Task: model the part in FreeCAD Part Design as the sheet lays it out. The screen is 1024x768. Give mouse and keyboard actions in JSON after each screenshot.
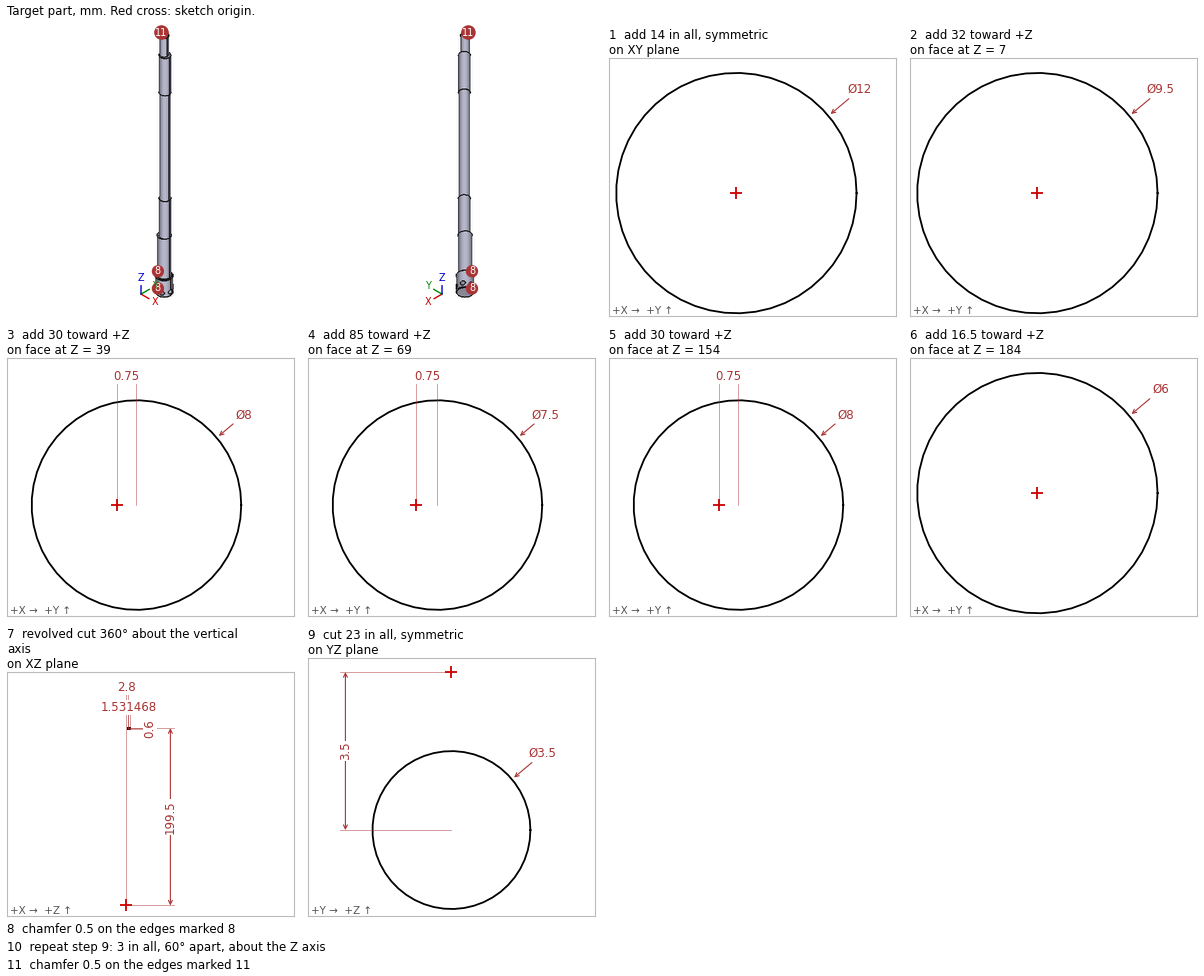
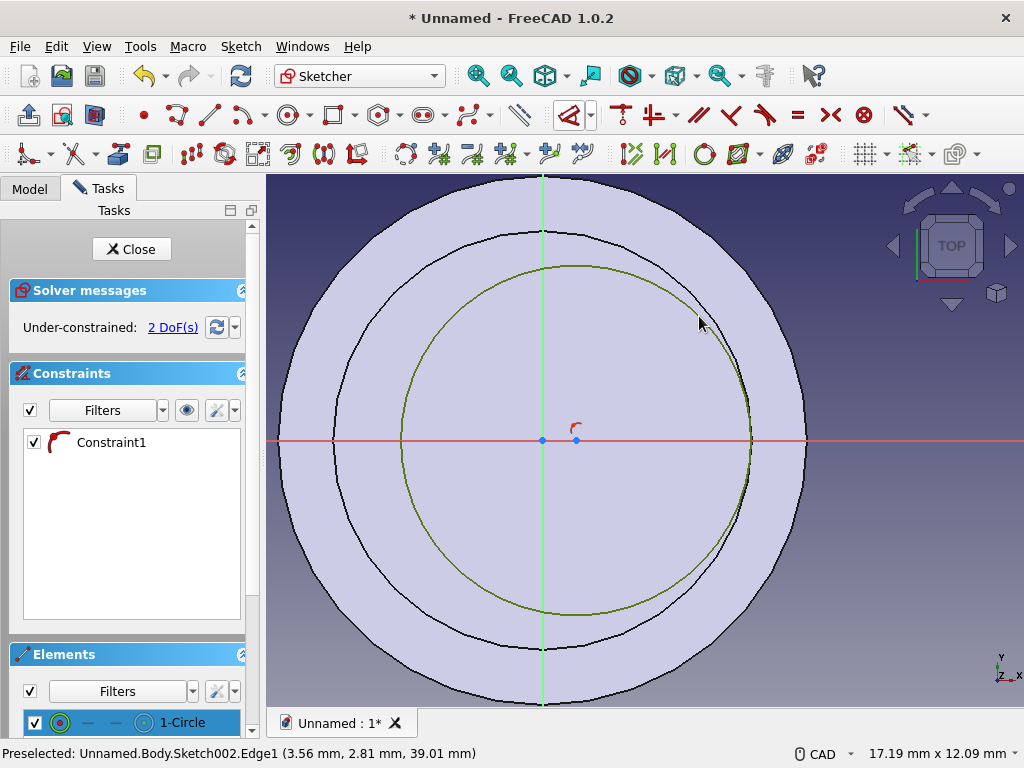
{"action": "key", "text": "k o"}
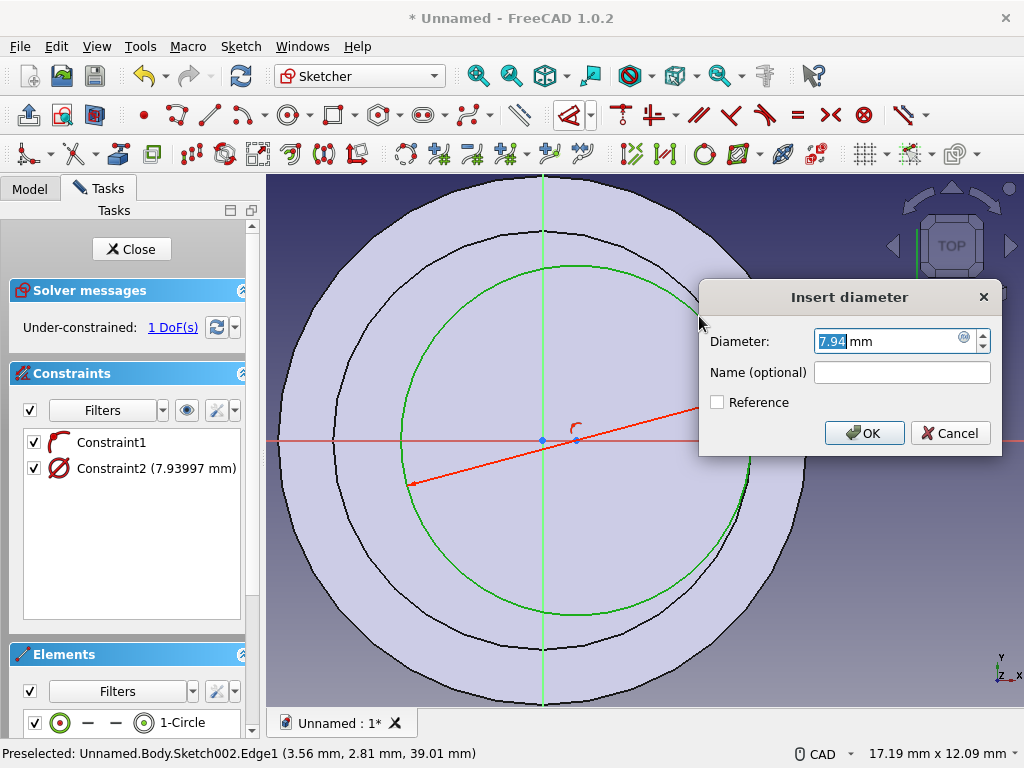
{"action": "type", "text": "8"}
{"action": "key", "text": "Return"}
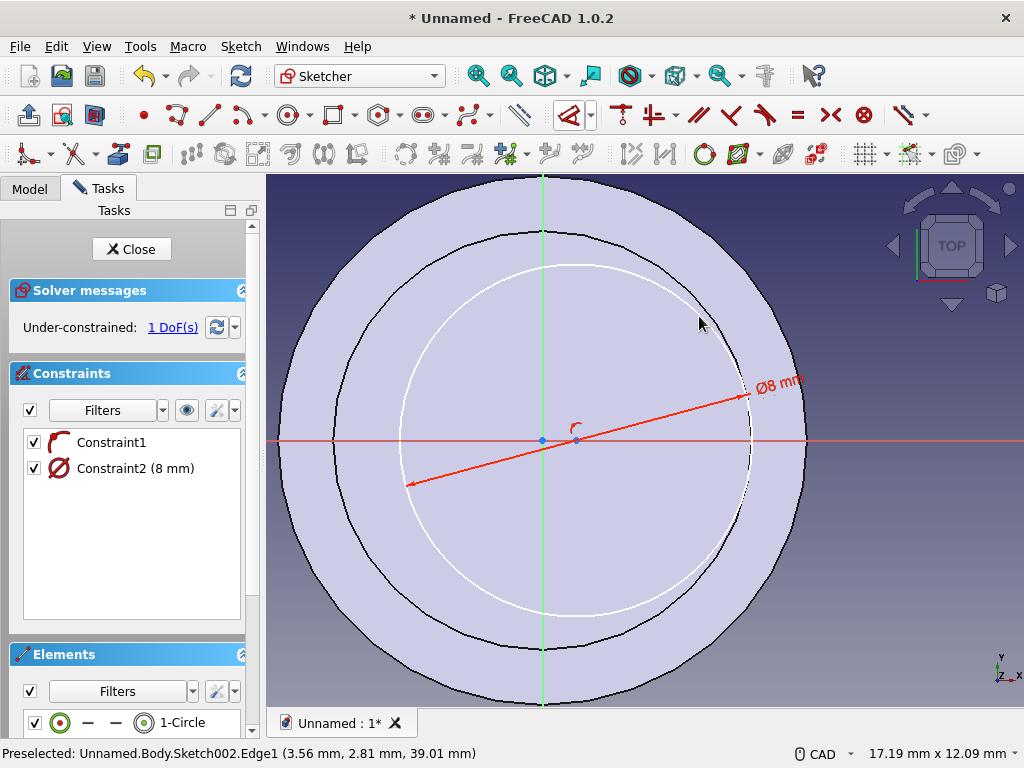
{"action": "left_click", "coordinate": [576, 440]}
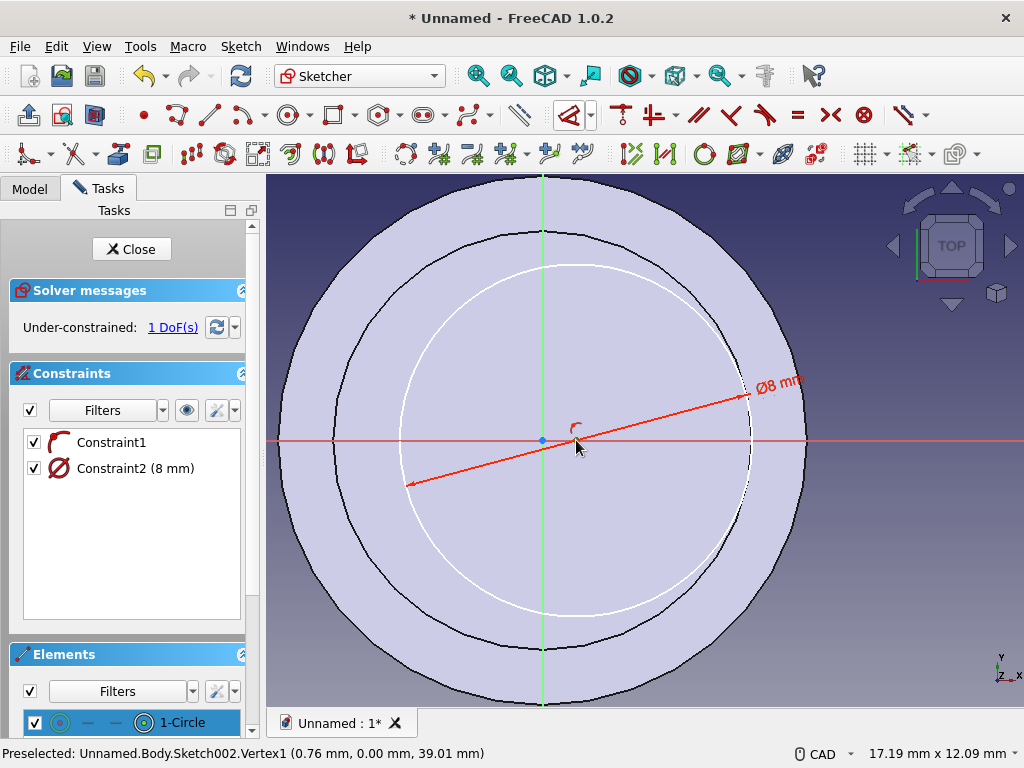
{"action": "key", "text": "l"}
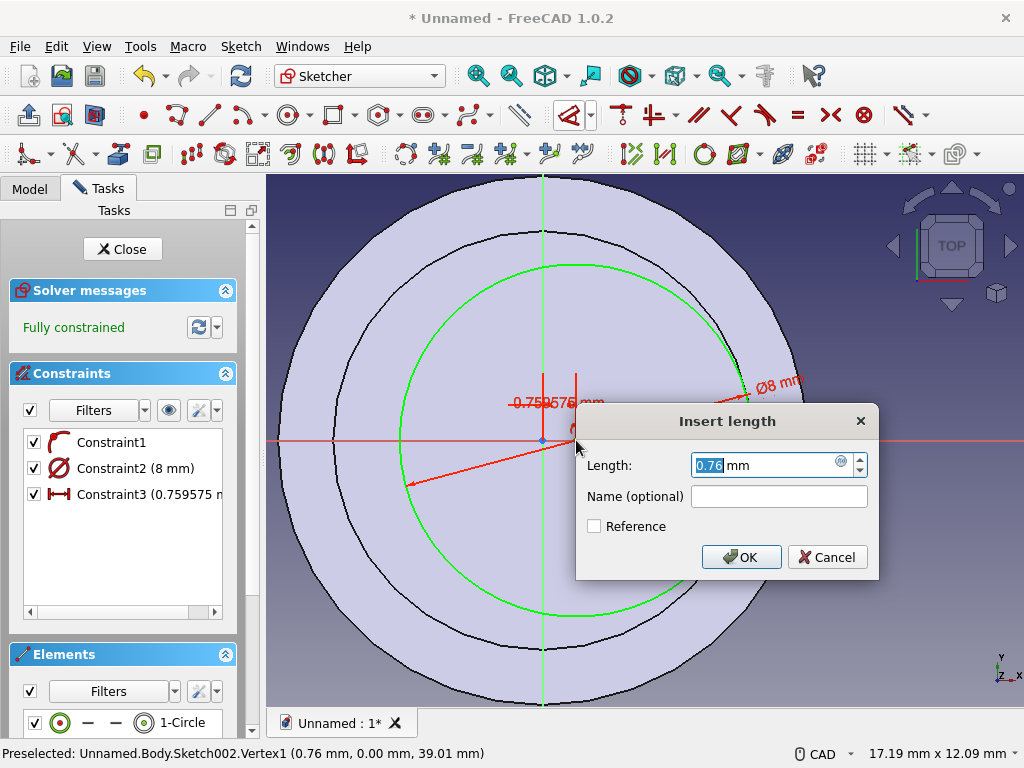
{"action": "type", "text": "0.75"}
{"action": "key", "text": "Return"}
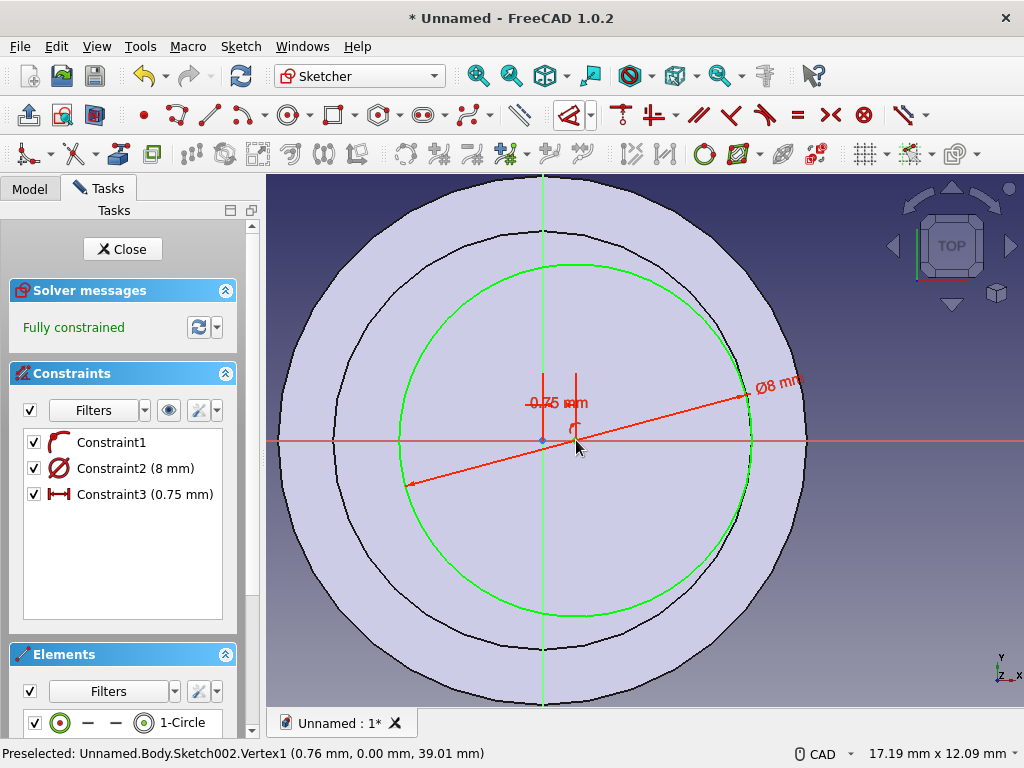
{"action": "left_click", "coordinate": [123, 249]}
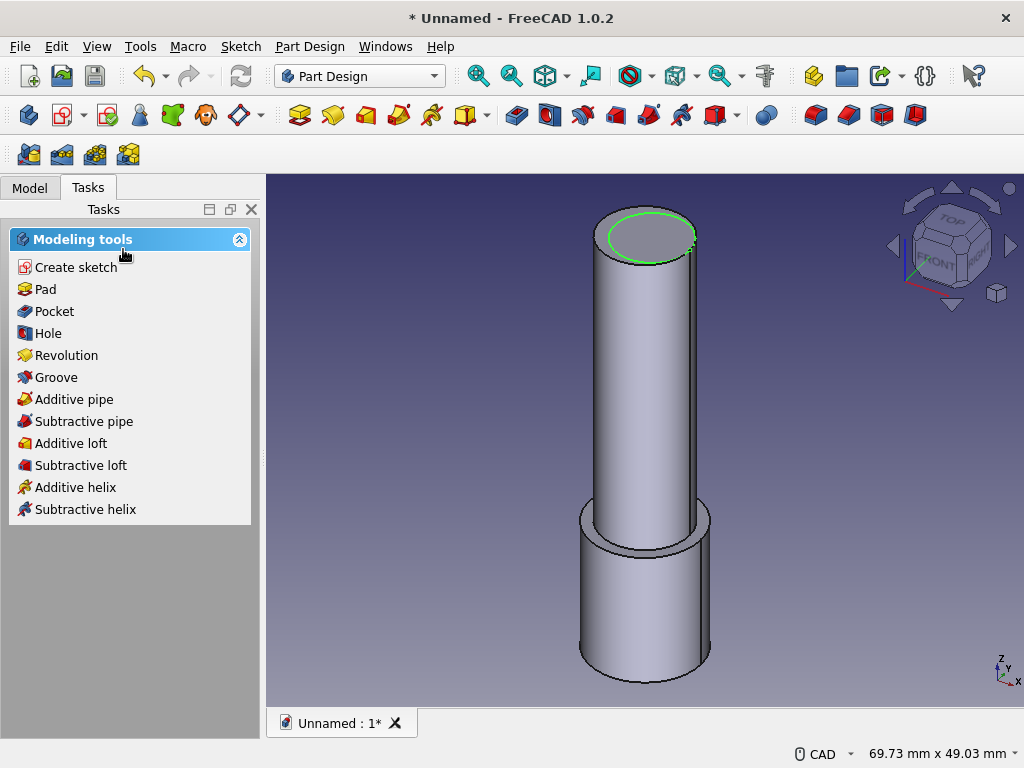
{"action": "left_click", "coordinate": [300, 116]}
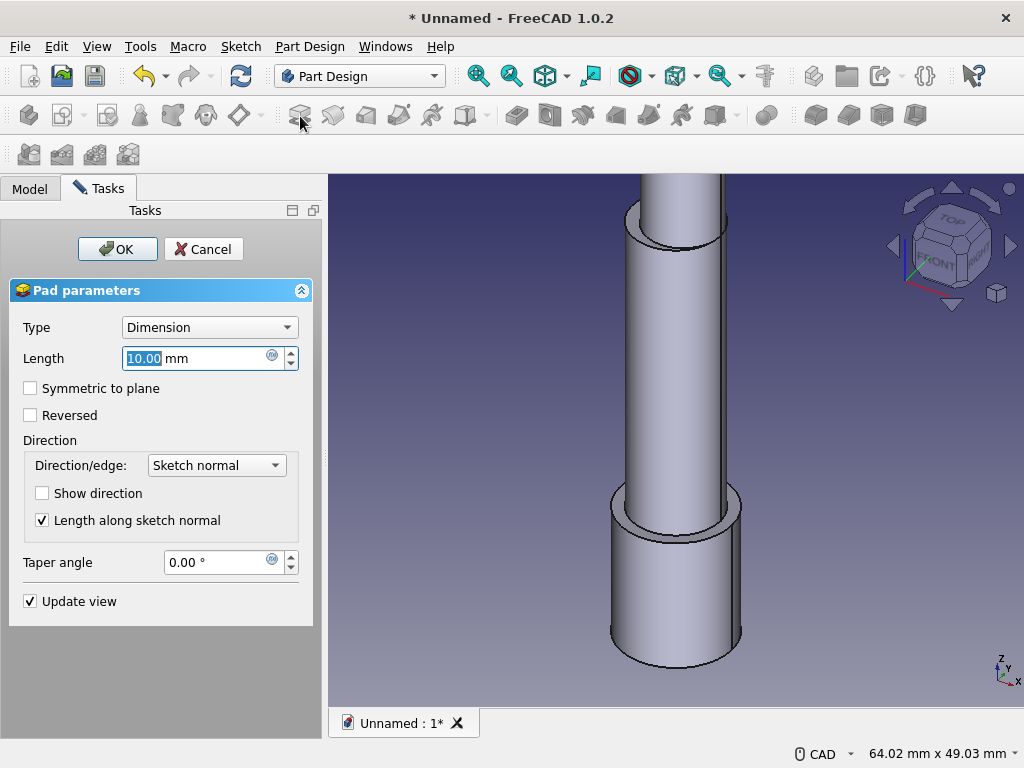
{"action": "type", "text": "30"}
{"action": "key", "text": "Tab"}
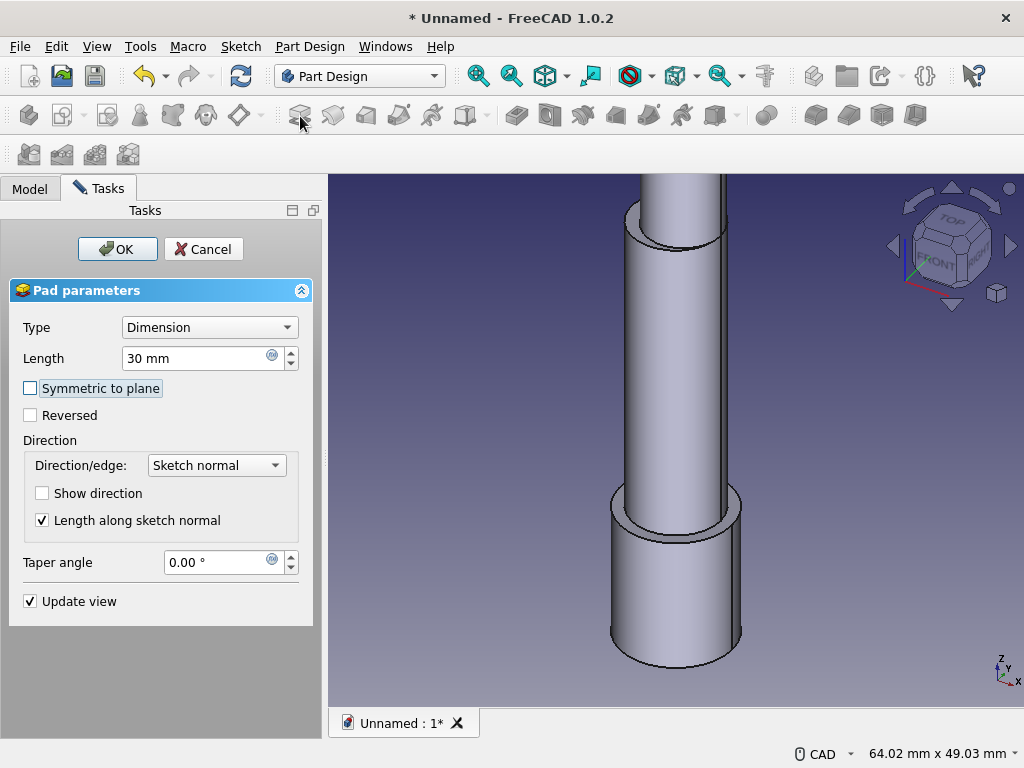
{"action": "left_click", "coordinate": [118, 249]}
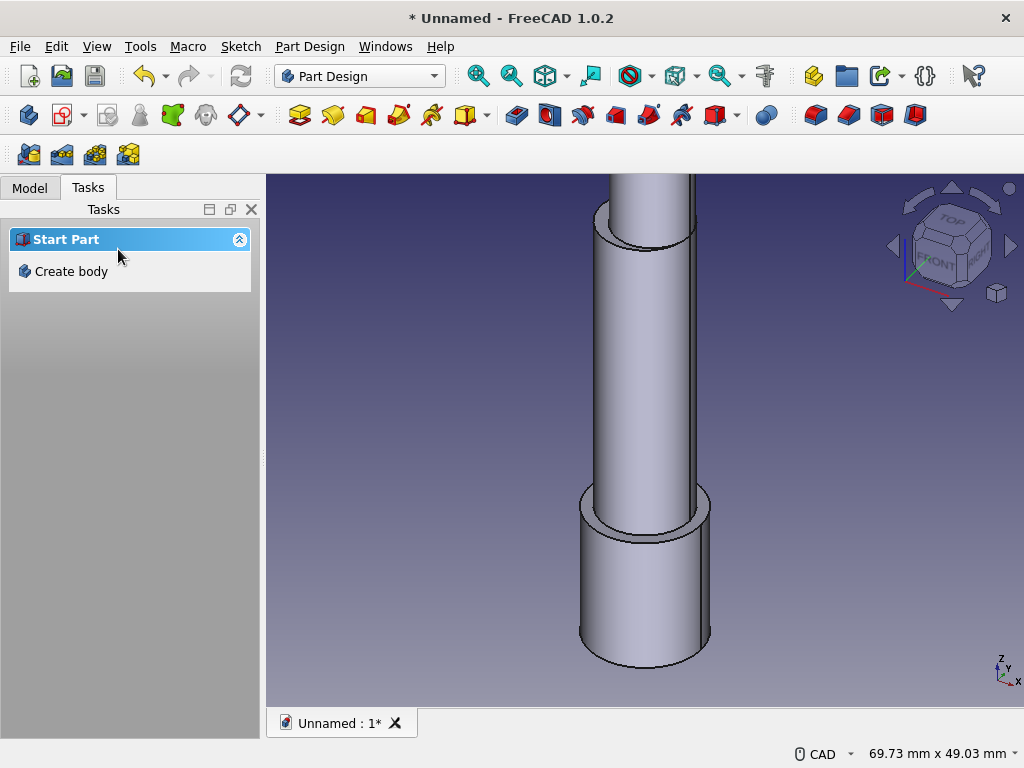
{"action": "key", "text": "v f"}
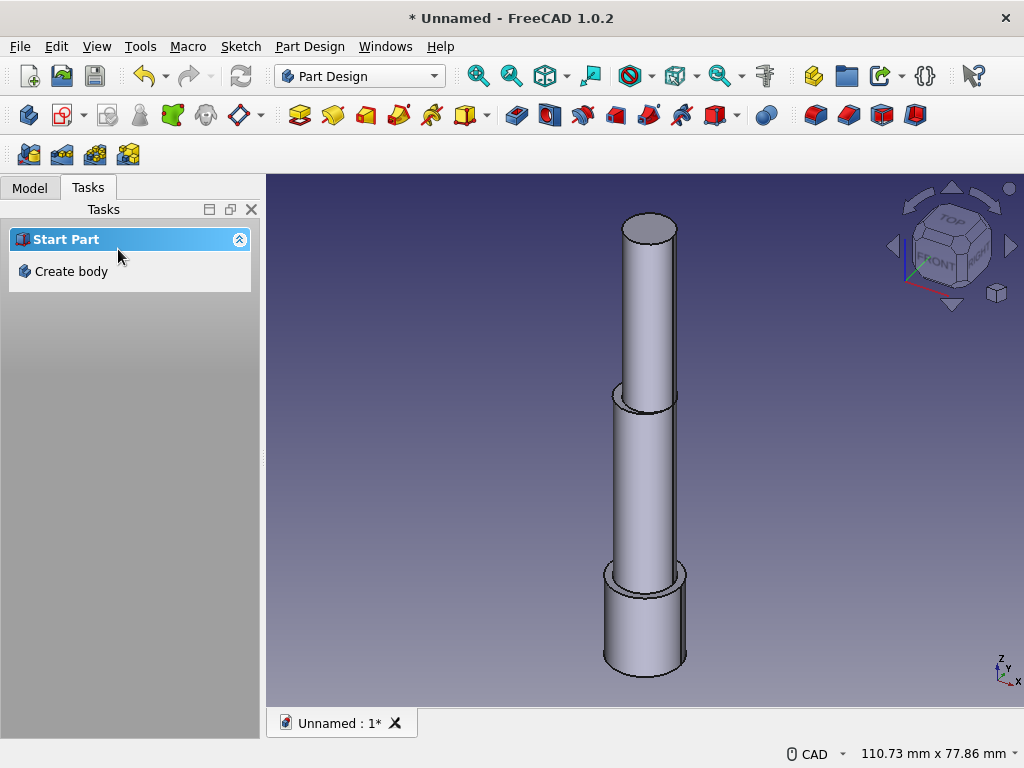
{"action": "left_click", "coordinate": [649, 228]}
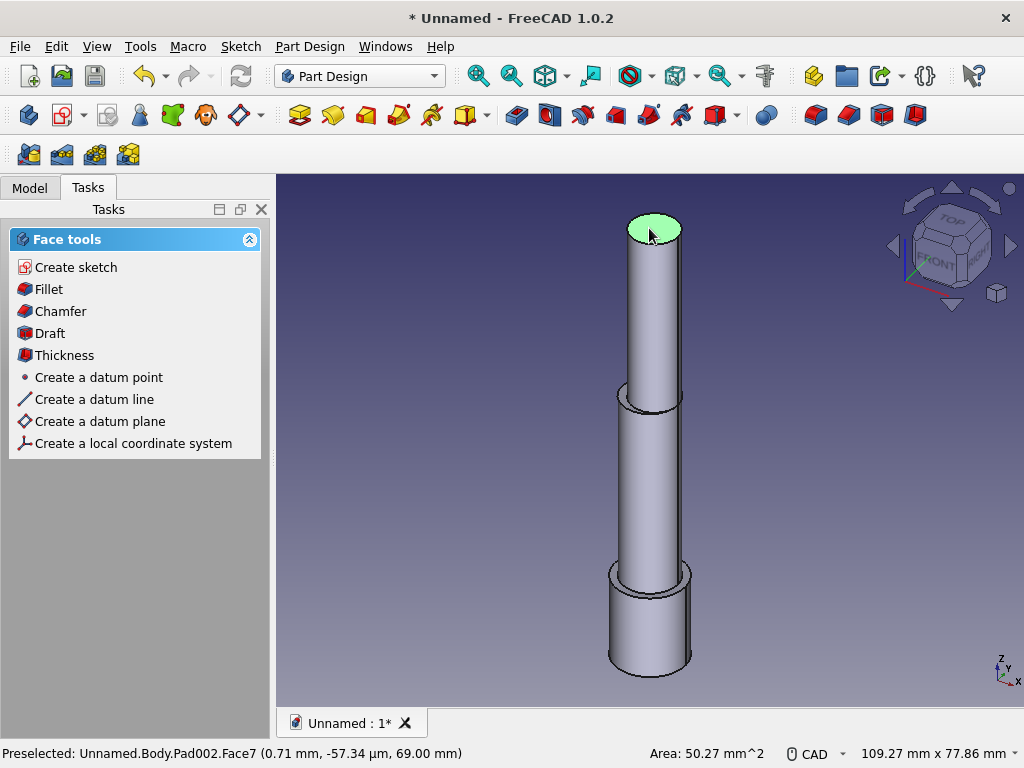
{"action": "left_click", "coordinate": [62, 116]}